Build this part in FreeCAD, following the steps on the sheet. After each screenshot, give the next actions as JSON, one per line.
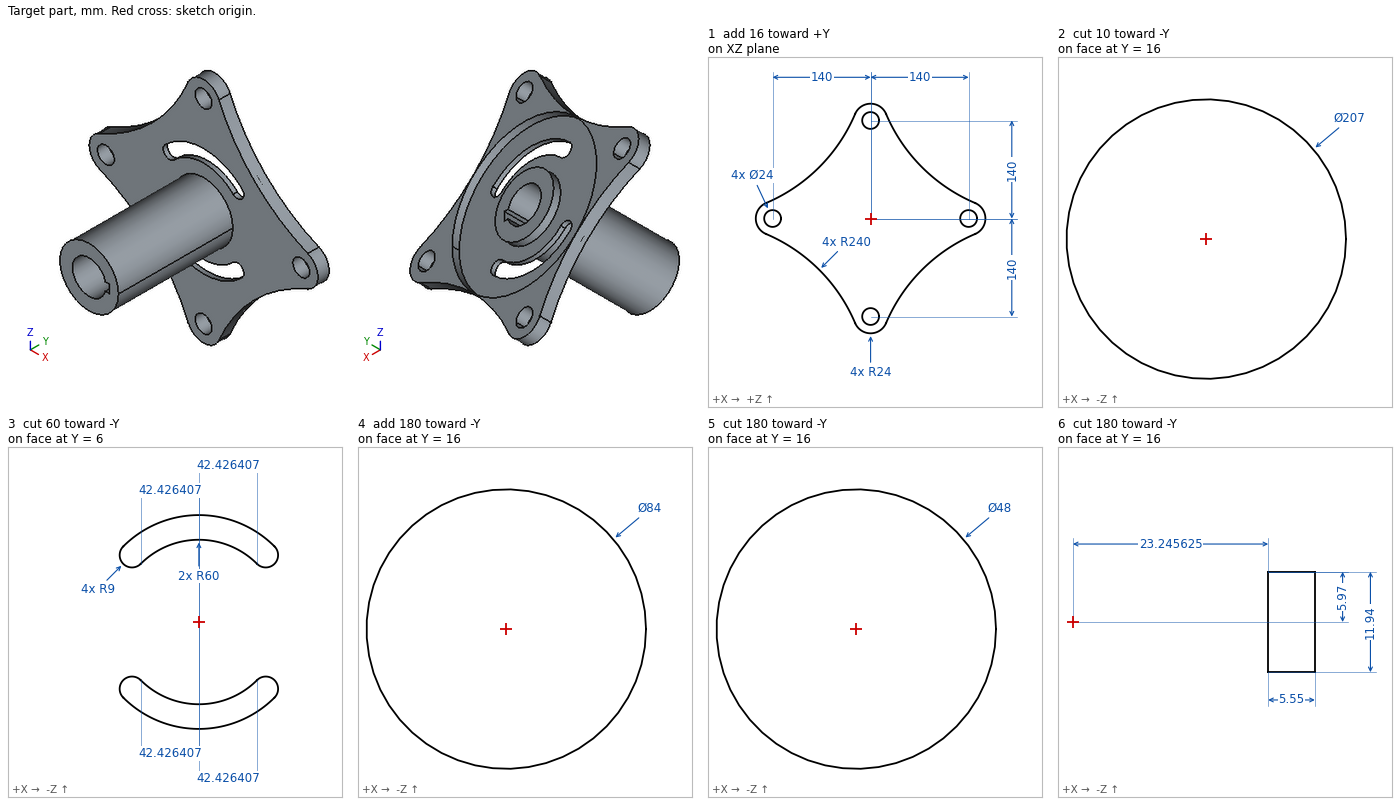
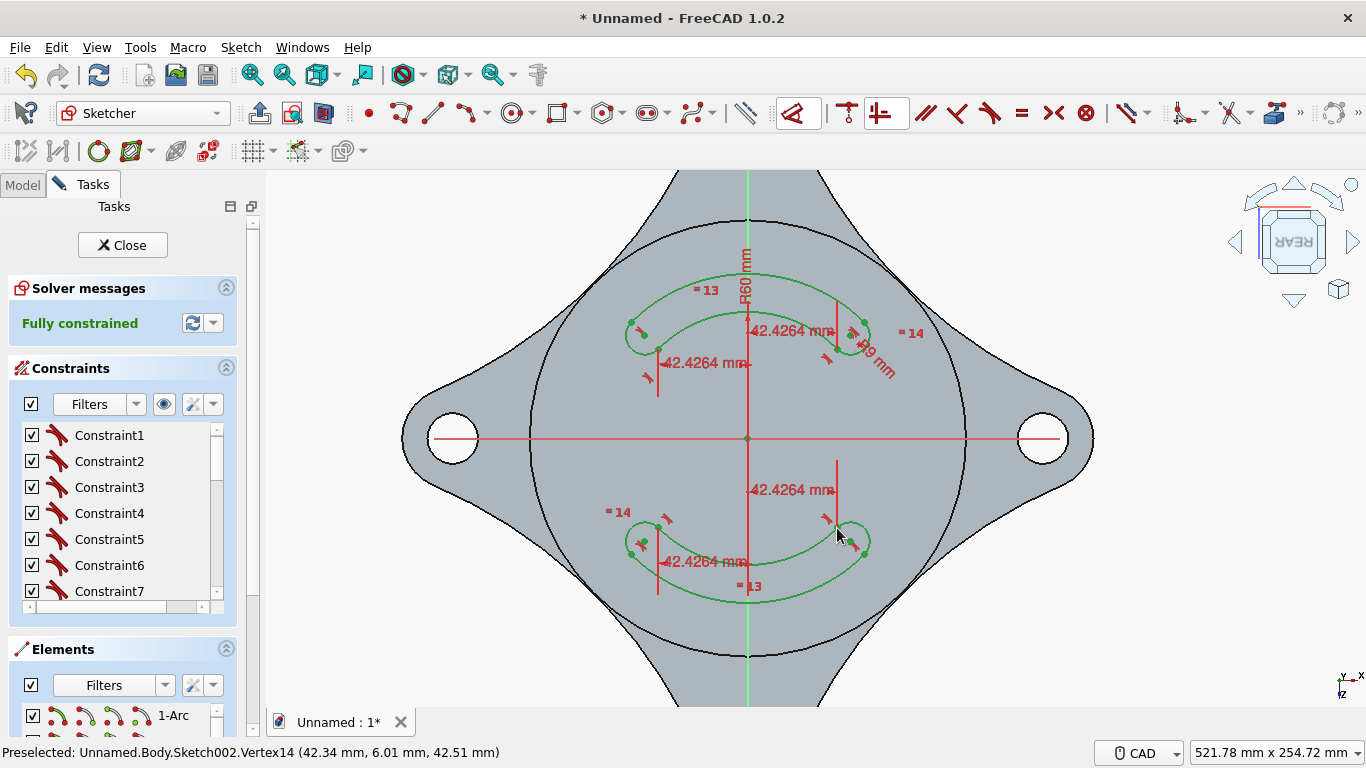
{"action": "left_click", "coordinate": [123, 245]}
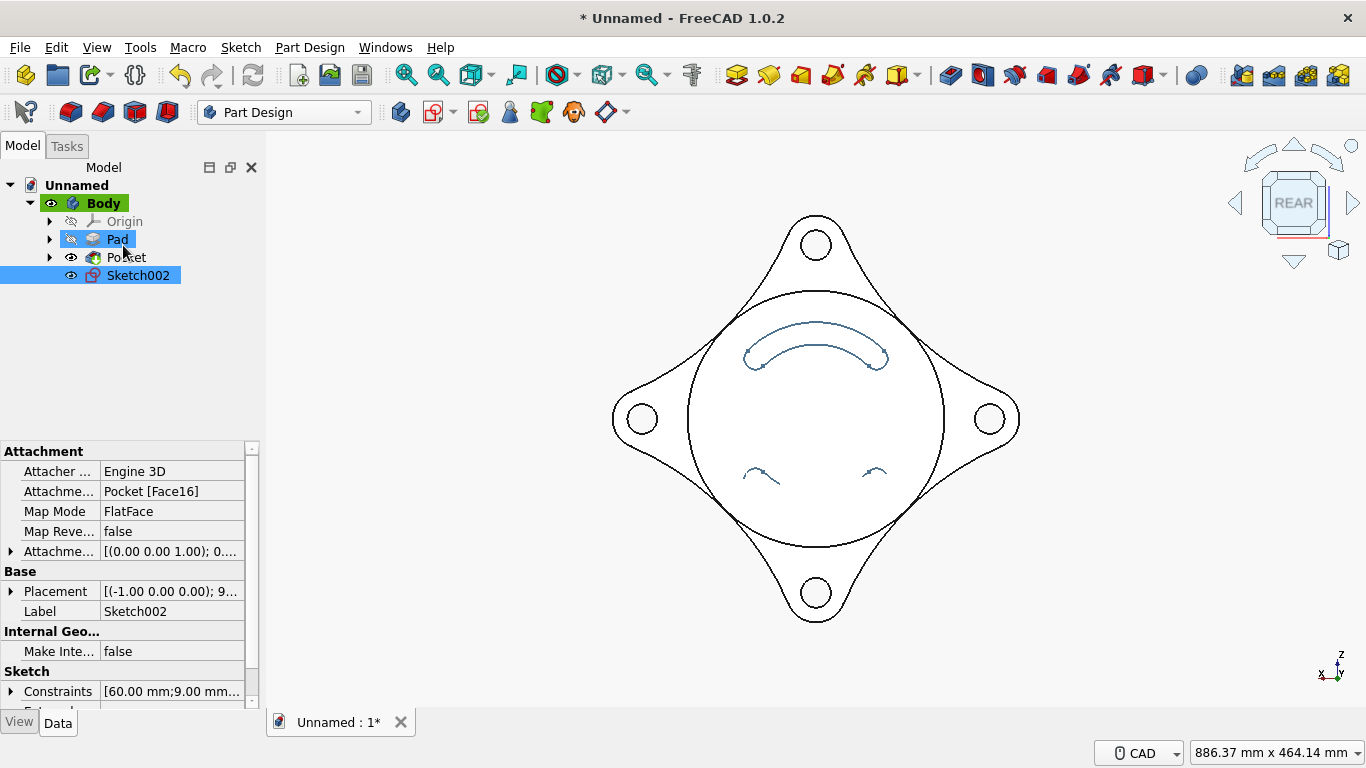
{"action": "left_click", "coordinate": [952, 76]}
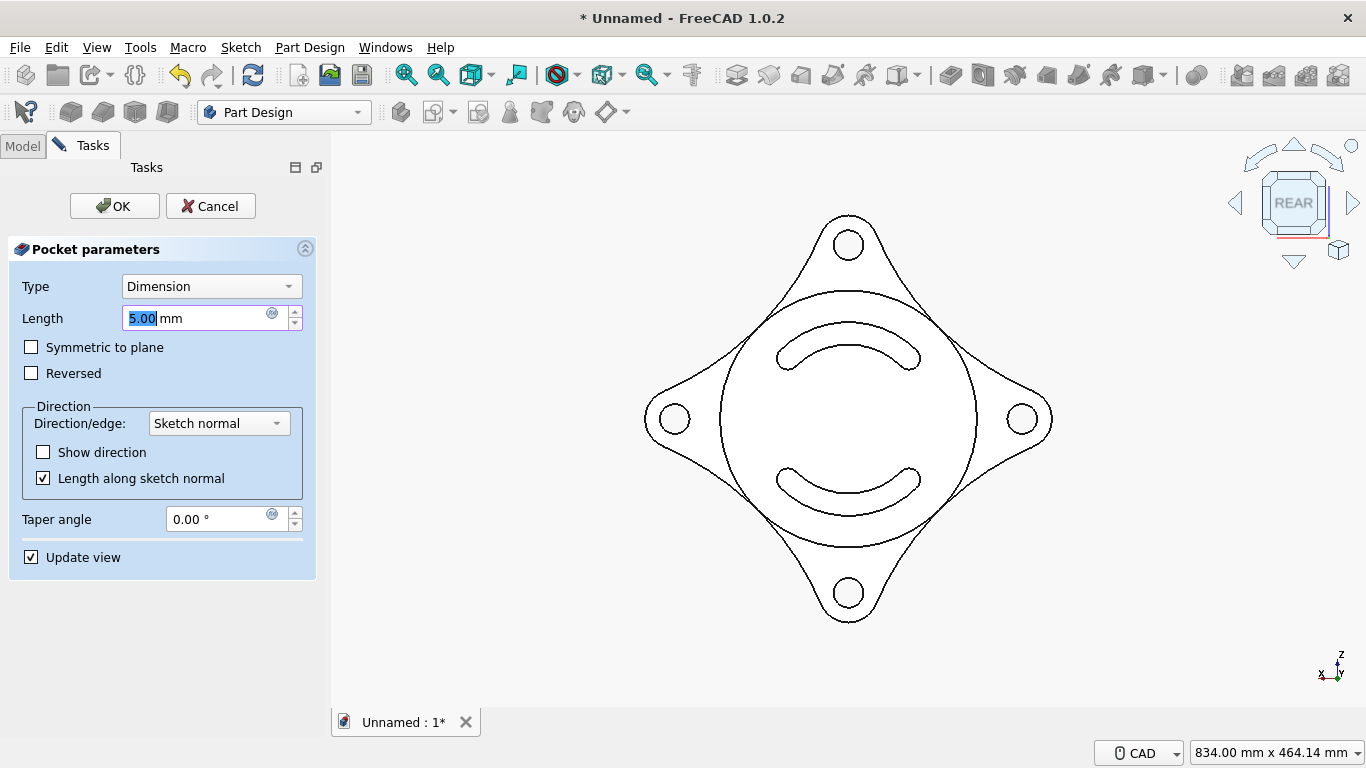
{"action": "type", "text": "60"}
{"action": "key", "text": "Tab"}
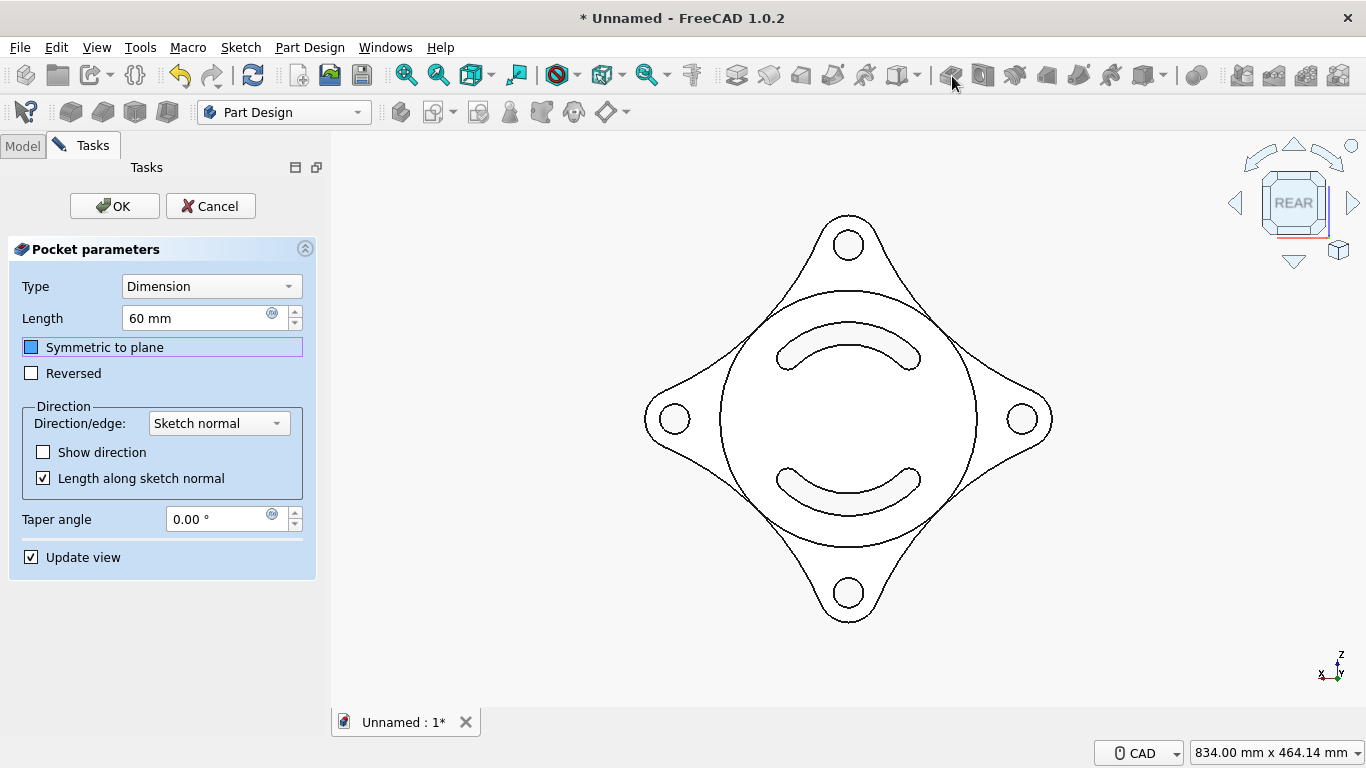
{"action": "left_click", "coordinate": [115, 206]}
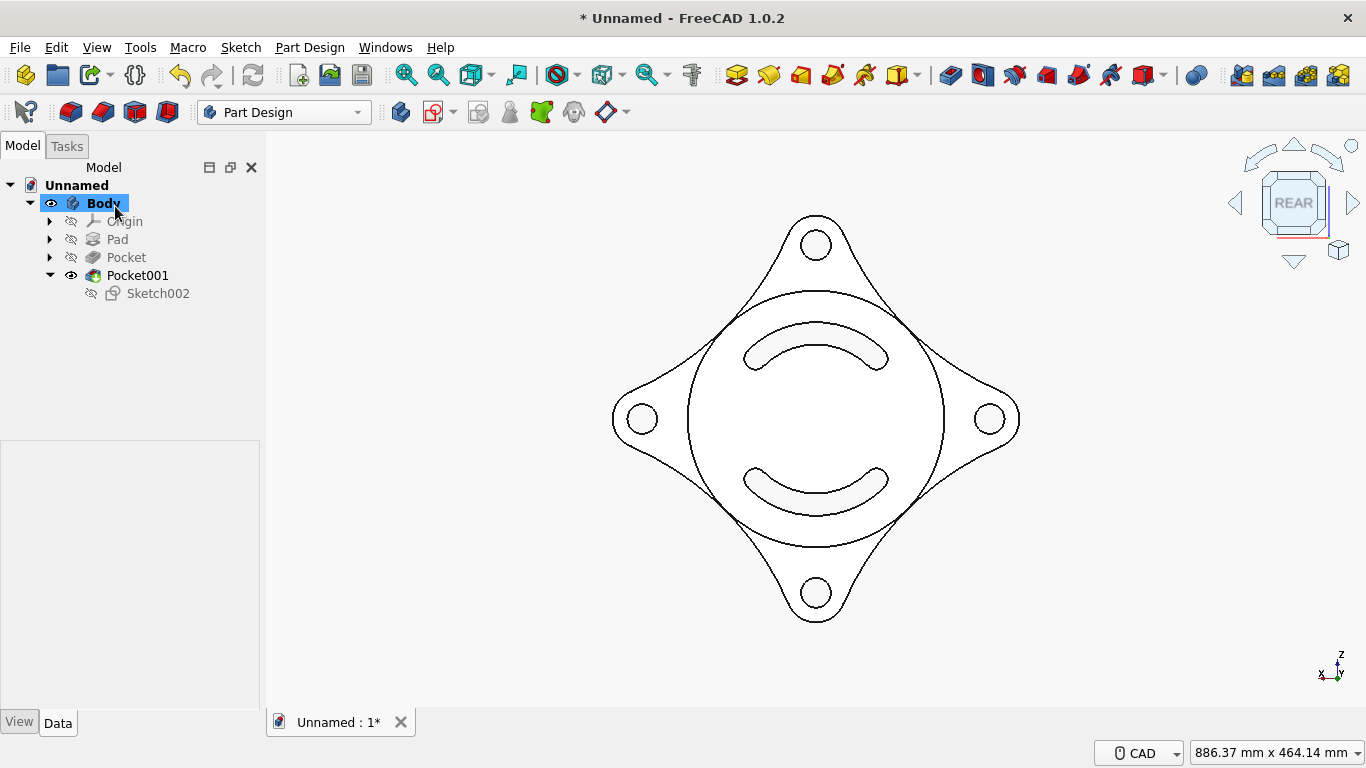
{"action": "scroll", "coordinate": [700, 476], "scroll_direction": "up", "scroll_amount": 11}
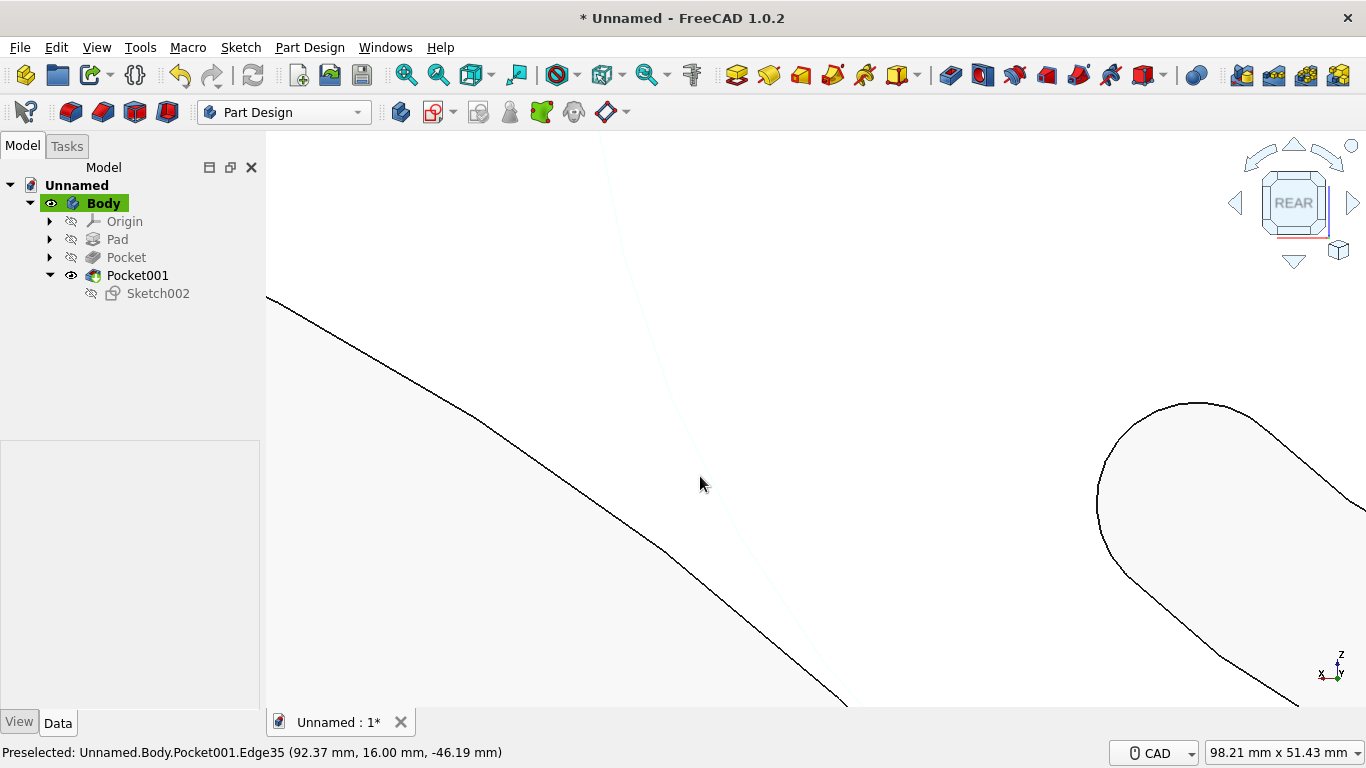
{"action": "left_click", "coordinate": [694, 481]}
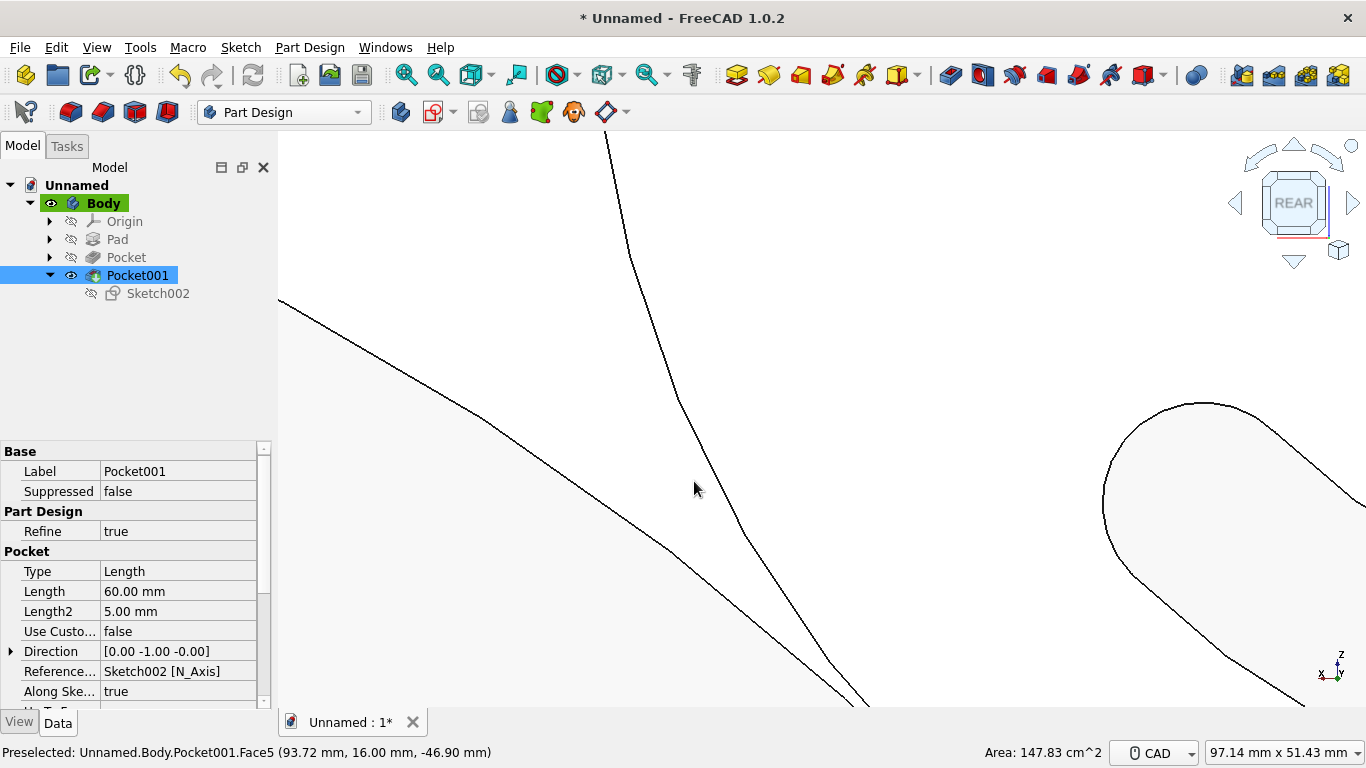
{"action": "left_click", "coordinate": [434, 112]}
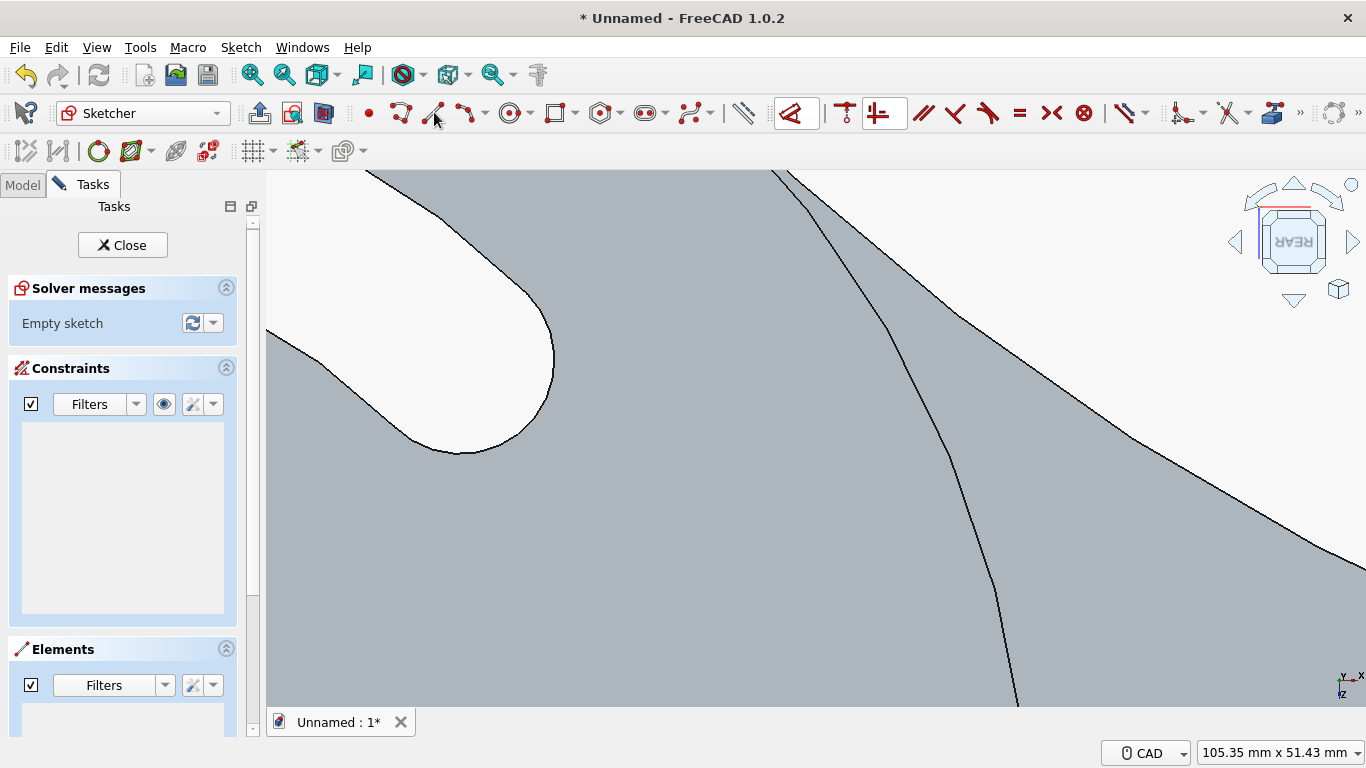
{"action": "scroll", "coordinate": [1201, 198], "scroll_direction": "down", "scroll_amount": 5}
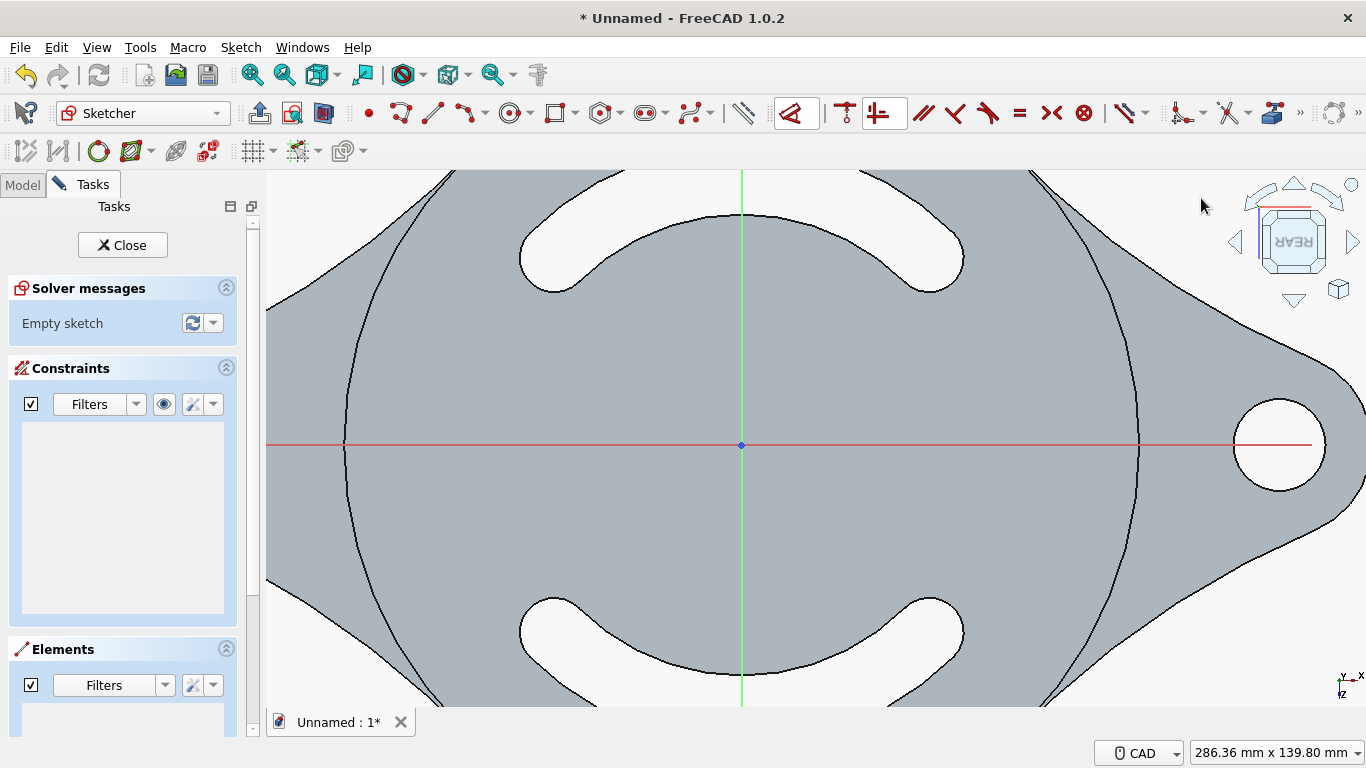
{"action": "left_click", "coordinate": [510, 114]}